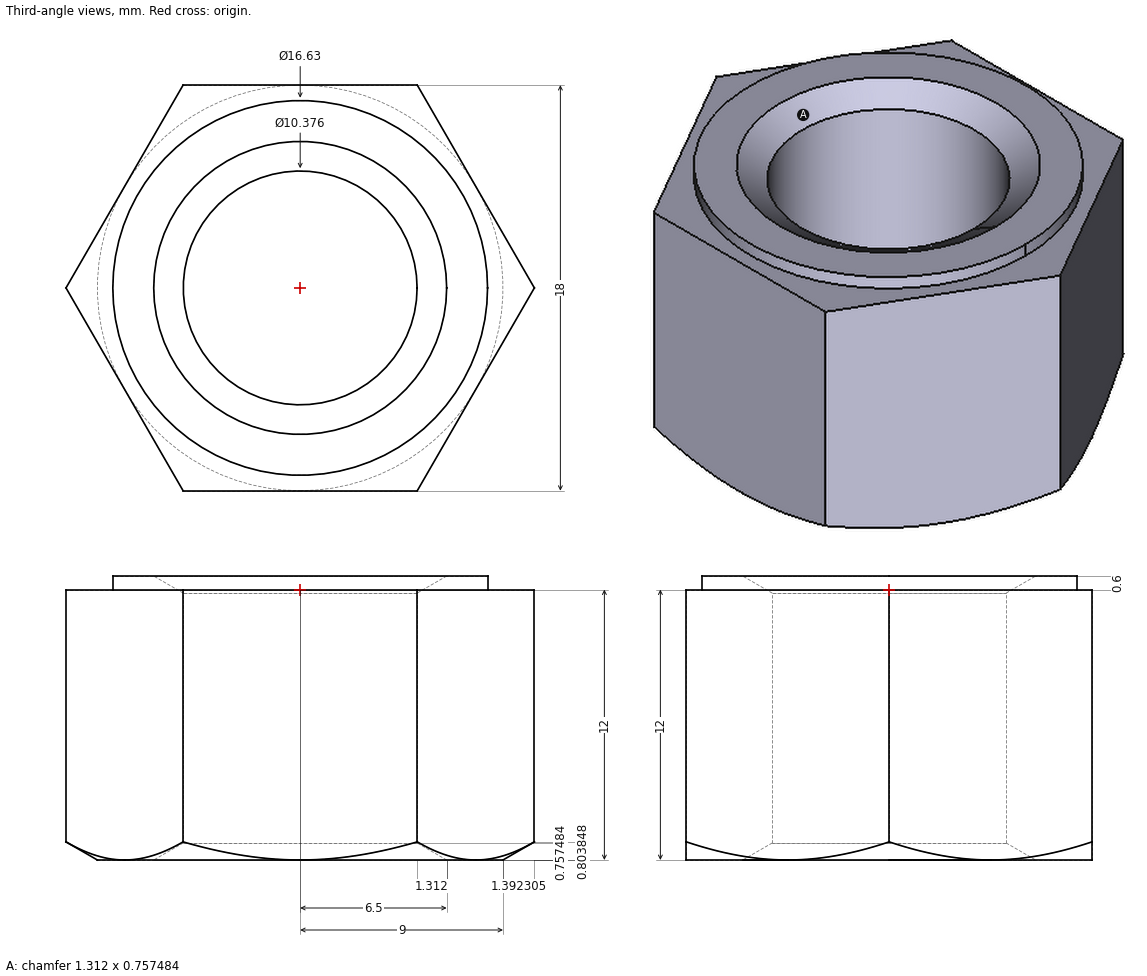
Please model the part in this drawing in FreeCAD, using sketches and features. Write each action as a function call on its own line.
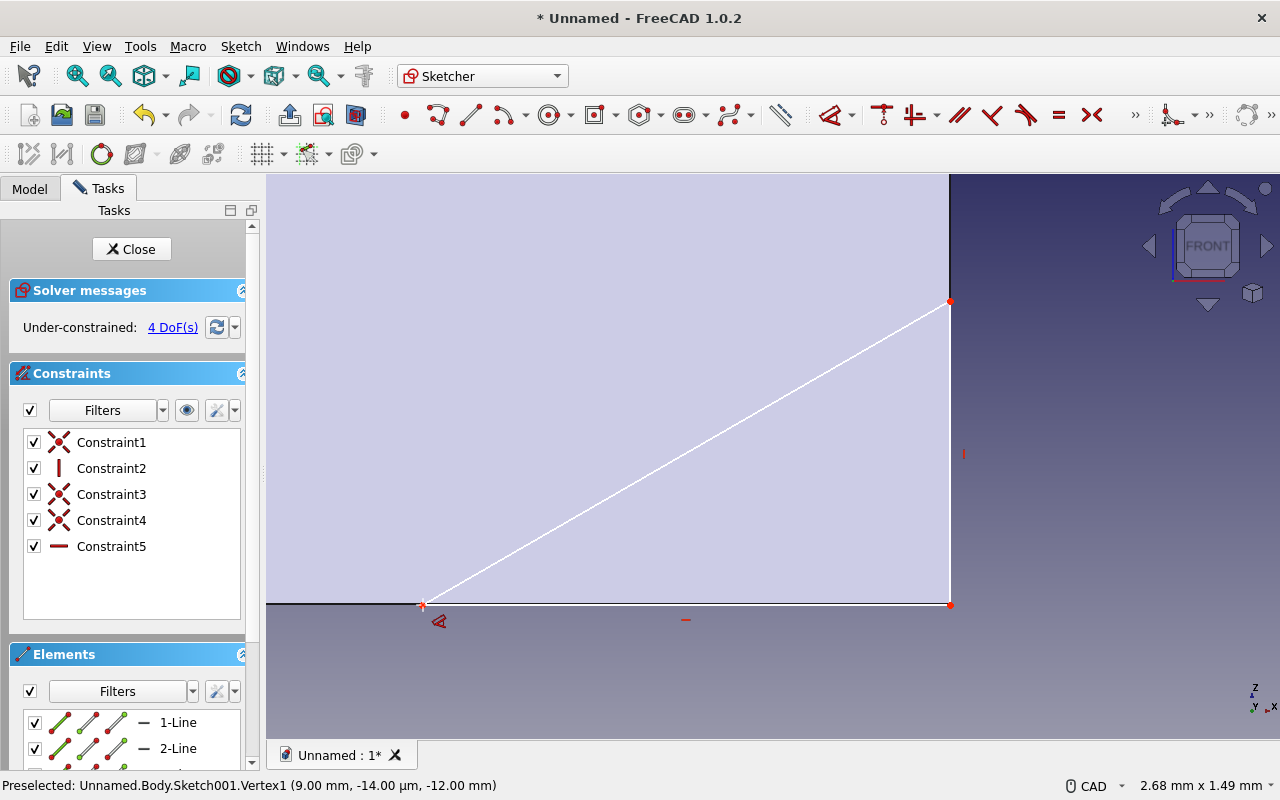
click(423, 605)
click(358, 639)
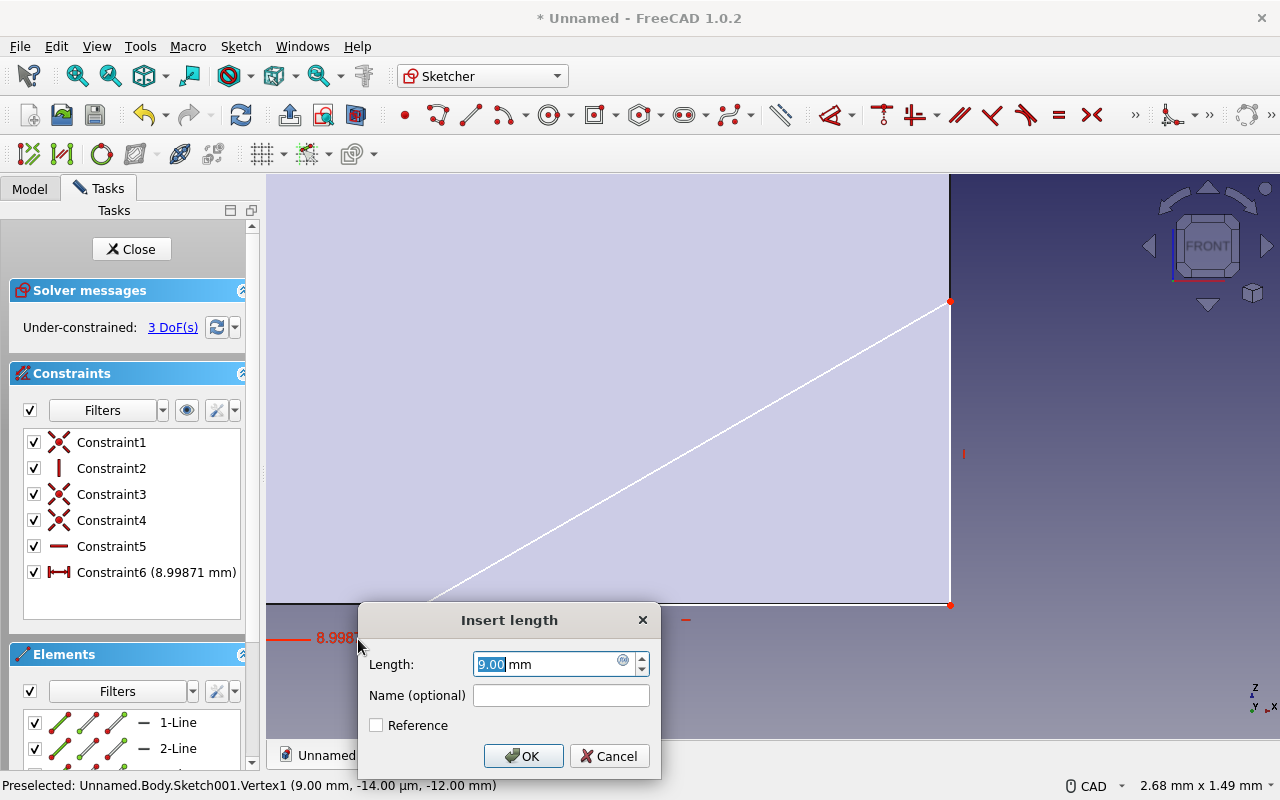
text(9)
key(Return)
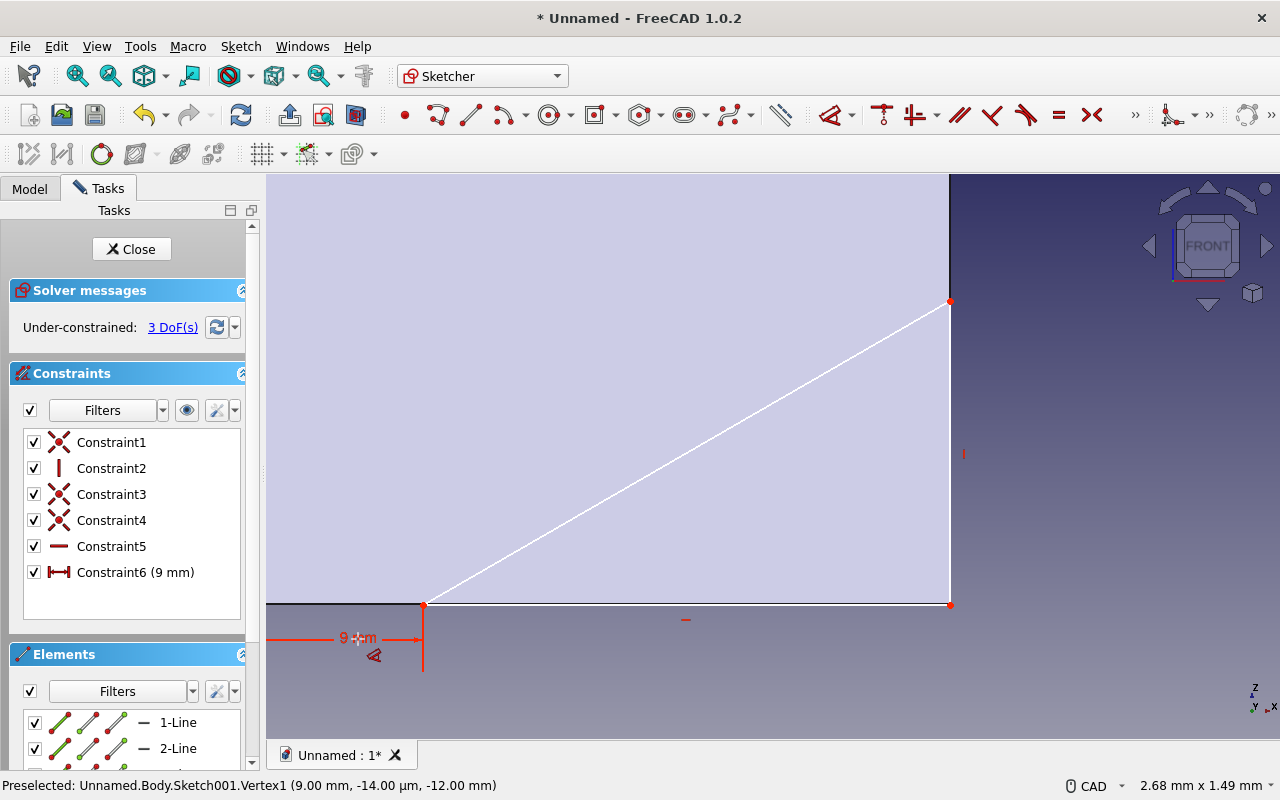
click(423, 605)
click(457, 403)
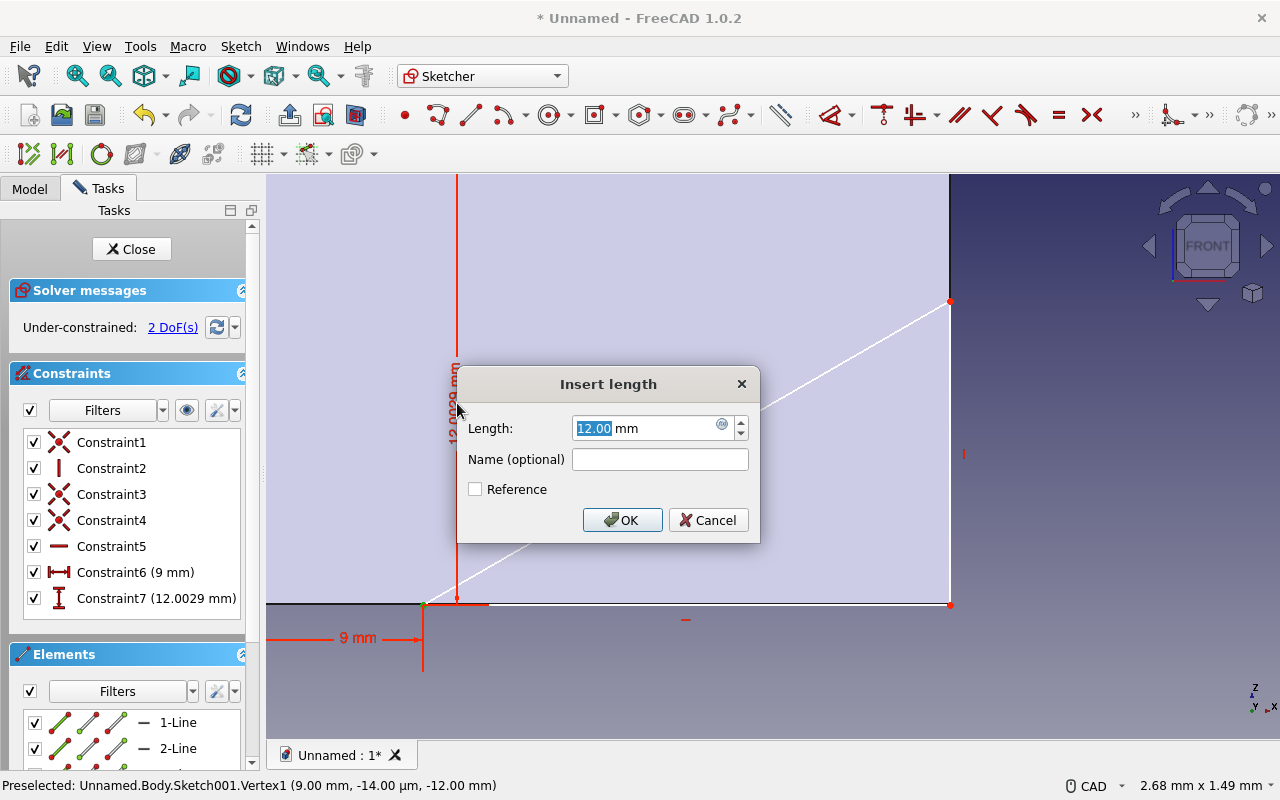
text(12)
key(Return)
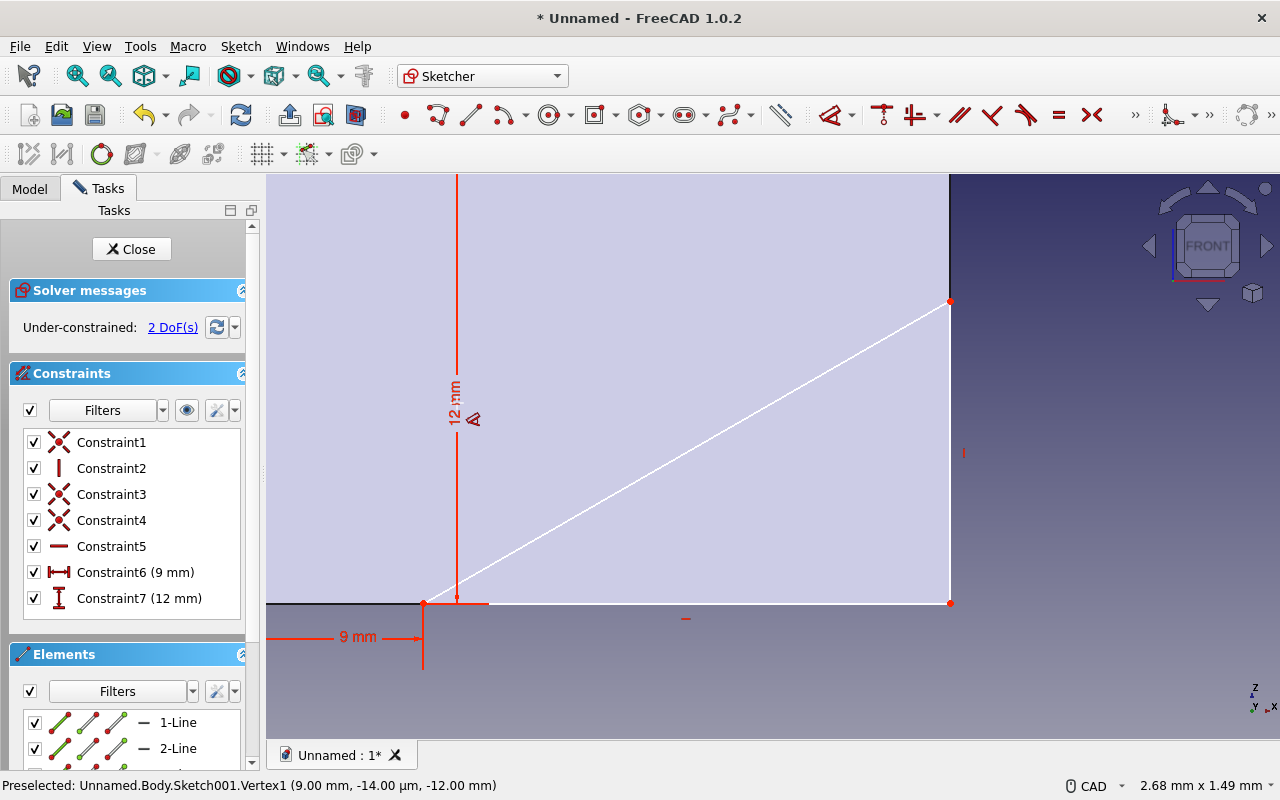
click(950, 392)
click(984, 452)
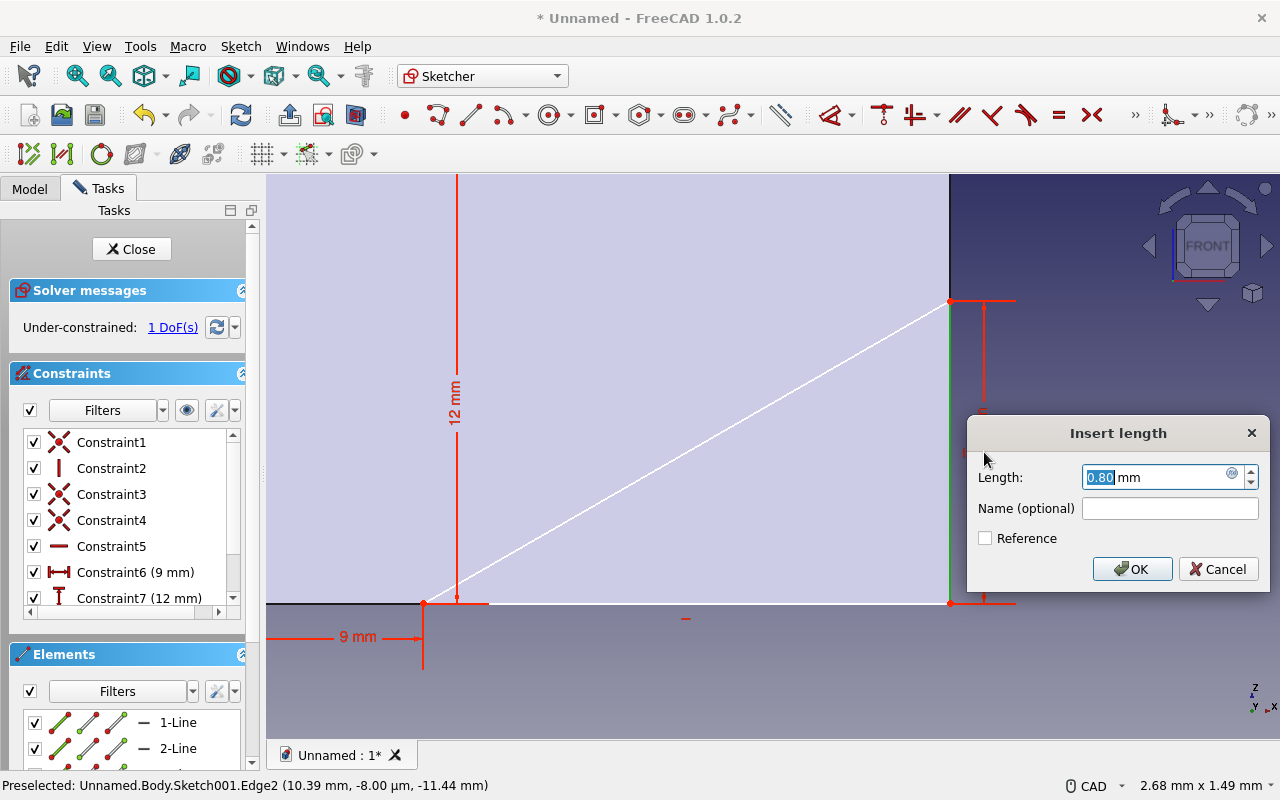
text(0.803848)
key(Return)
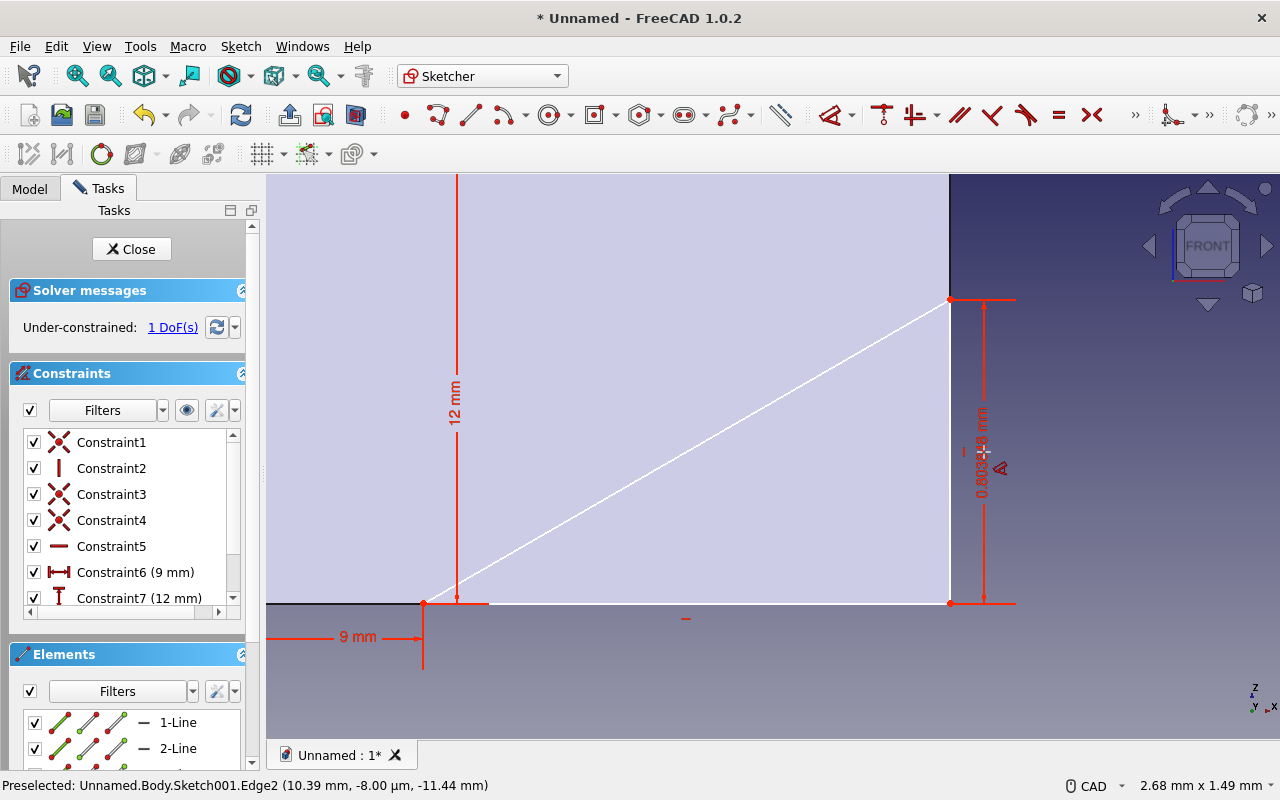
click(792, 604)
click(687, 638)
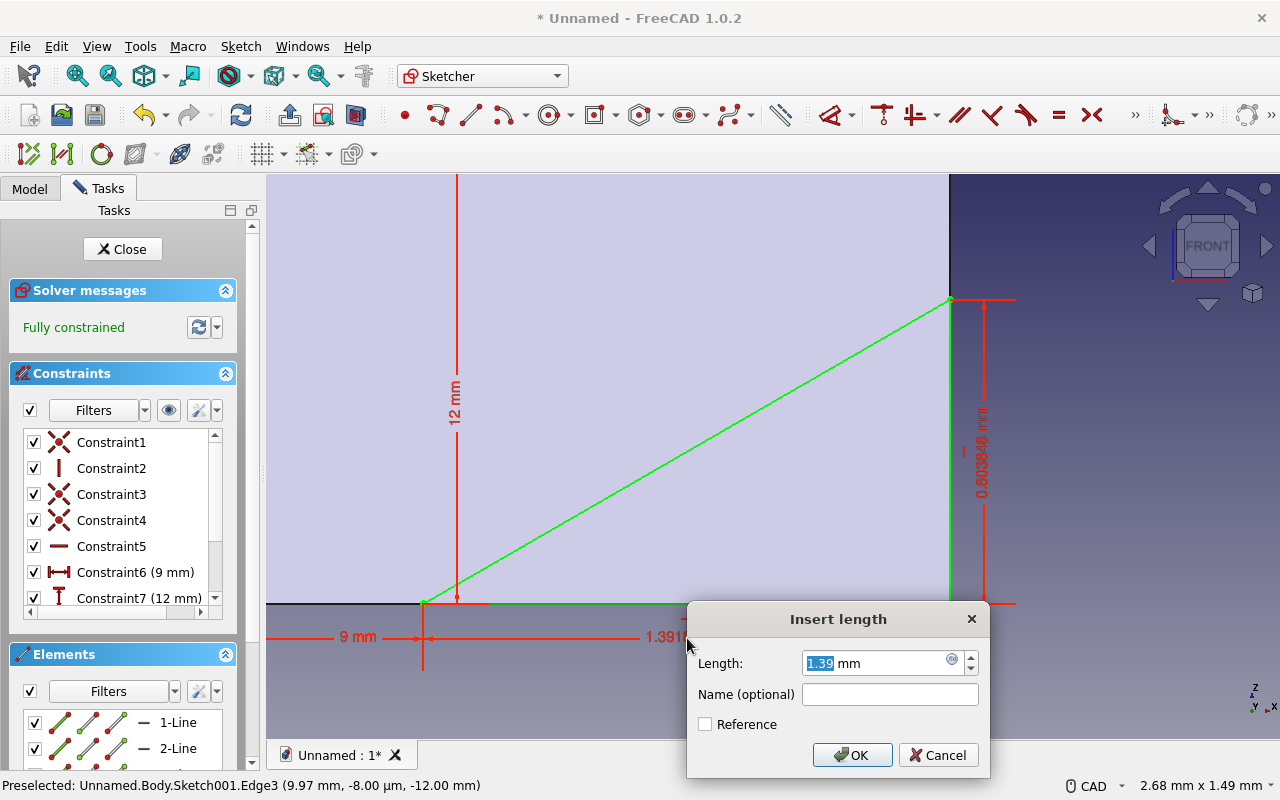
text(1.392305)
key(Return)
key(Escape)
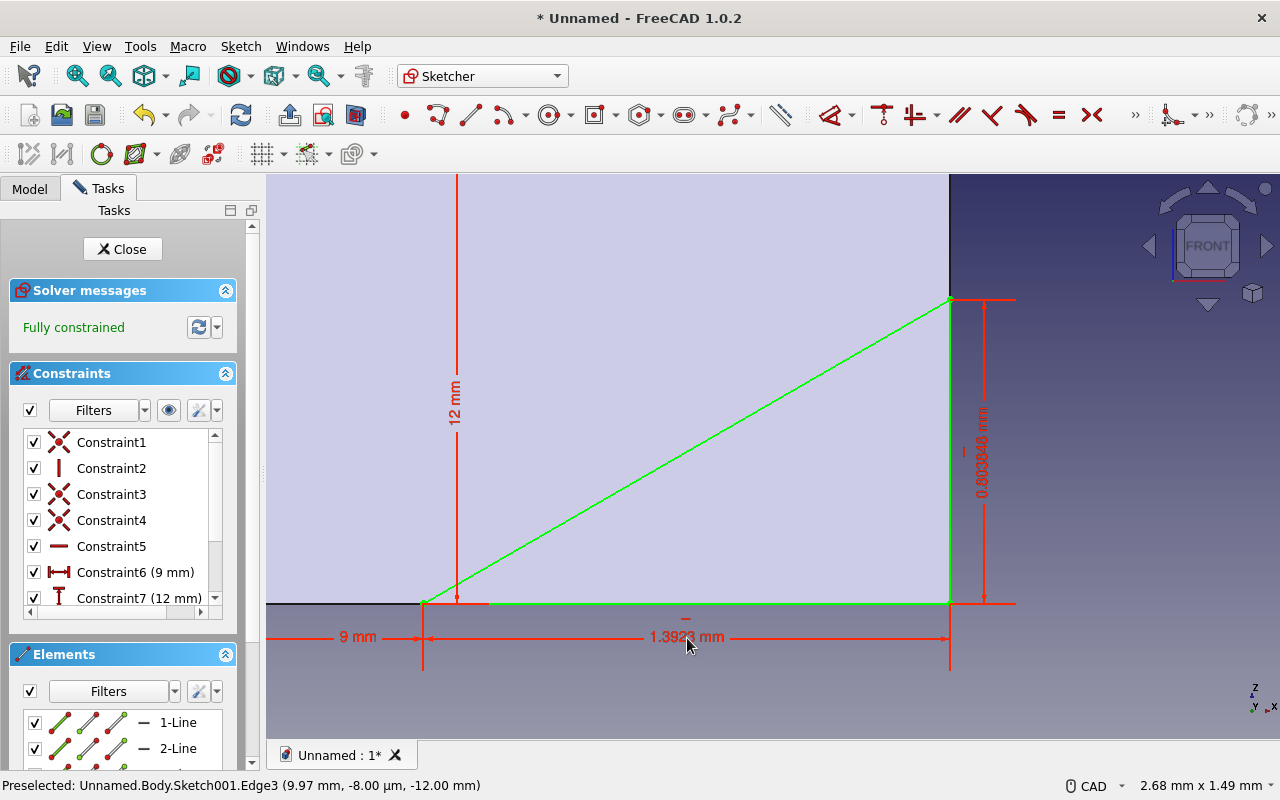
click(123, 249)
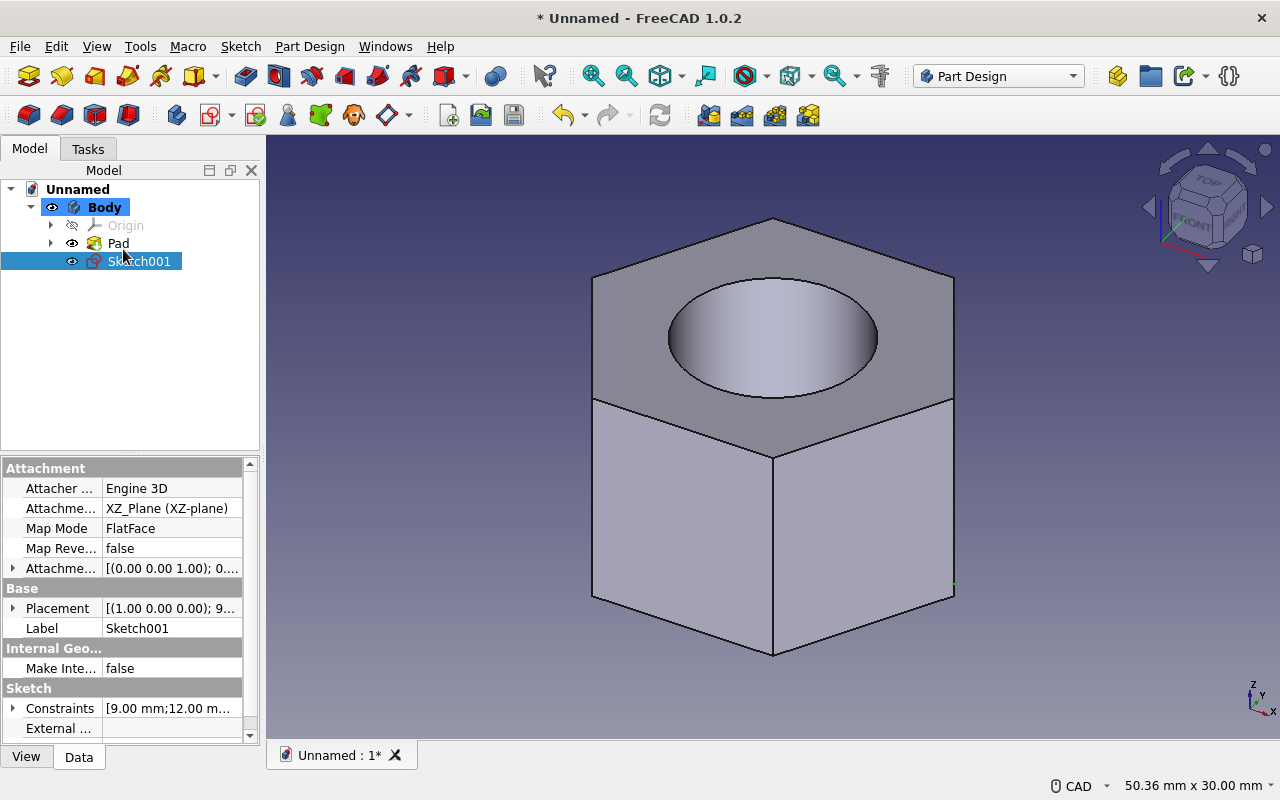
click(312, 76)